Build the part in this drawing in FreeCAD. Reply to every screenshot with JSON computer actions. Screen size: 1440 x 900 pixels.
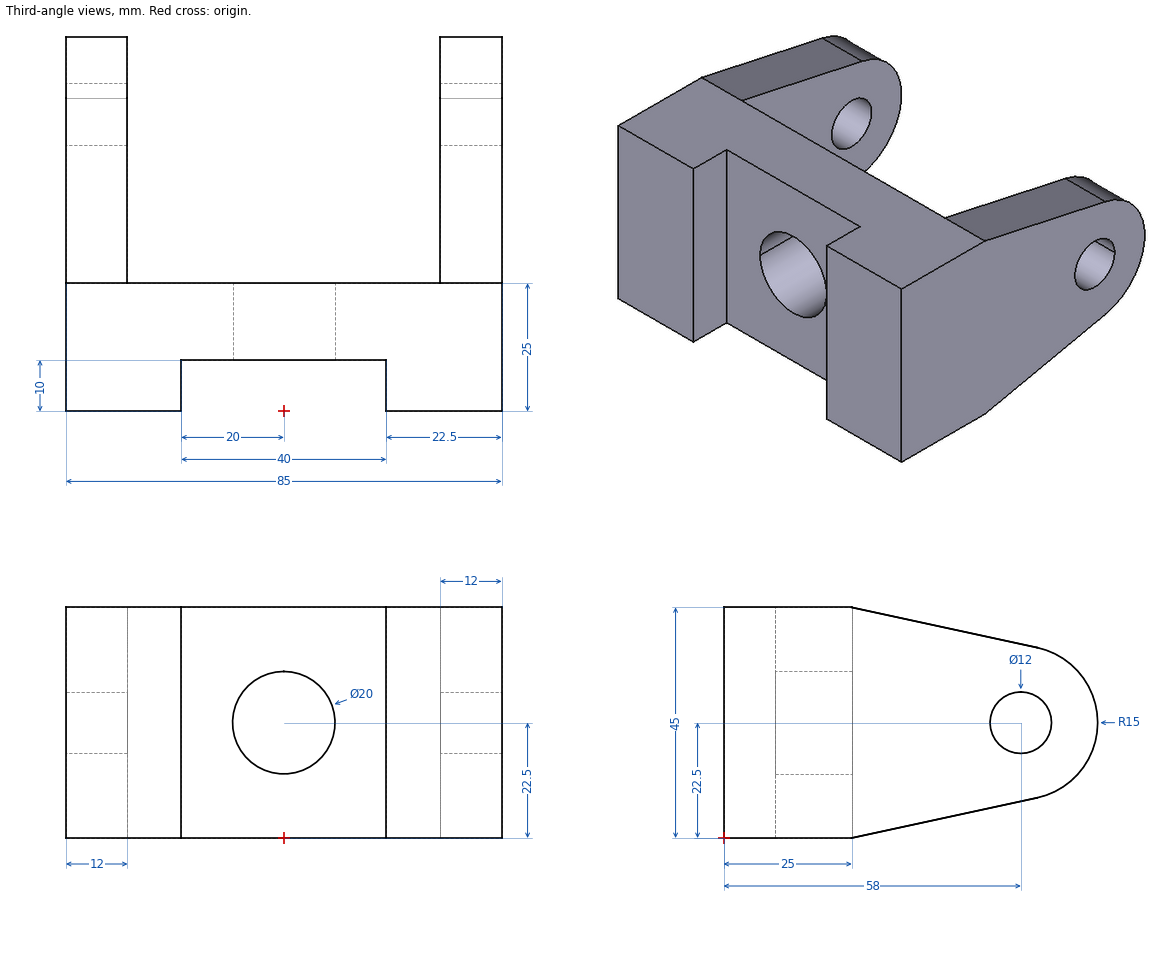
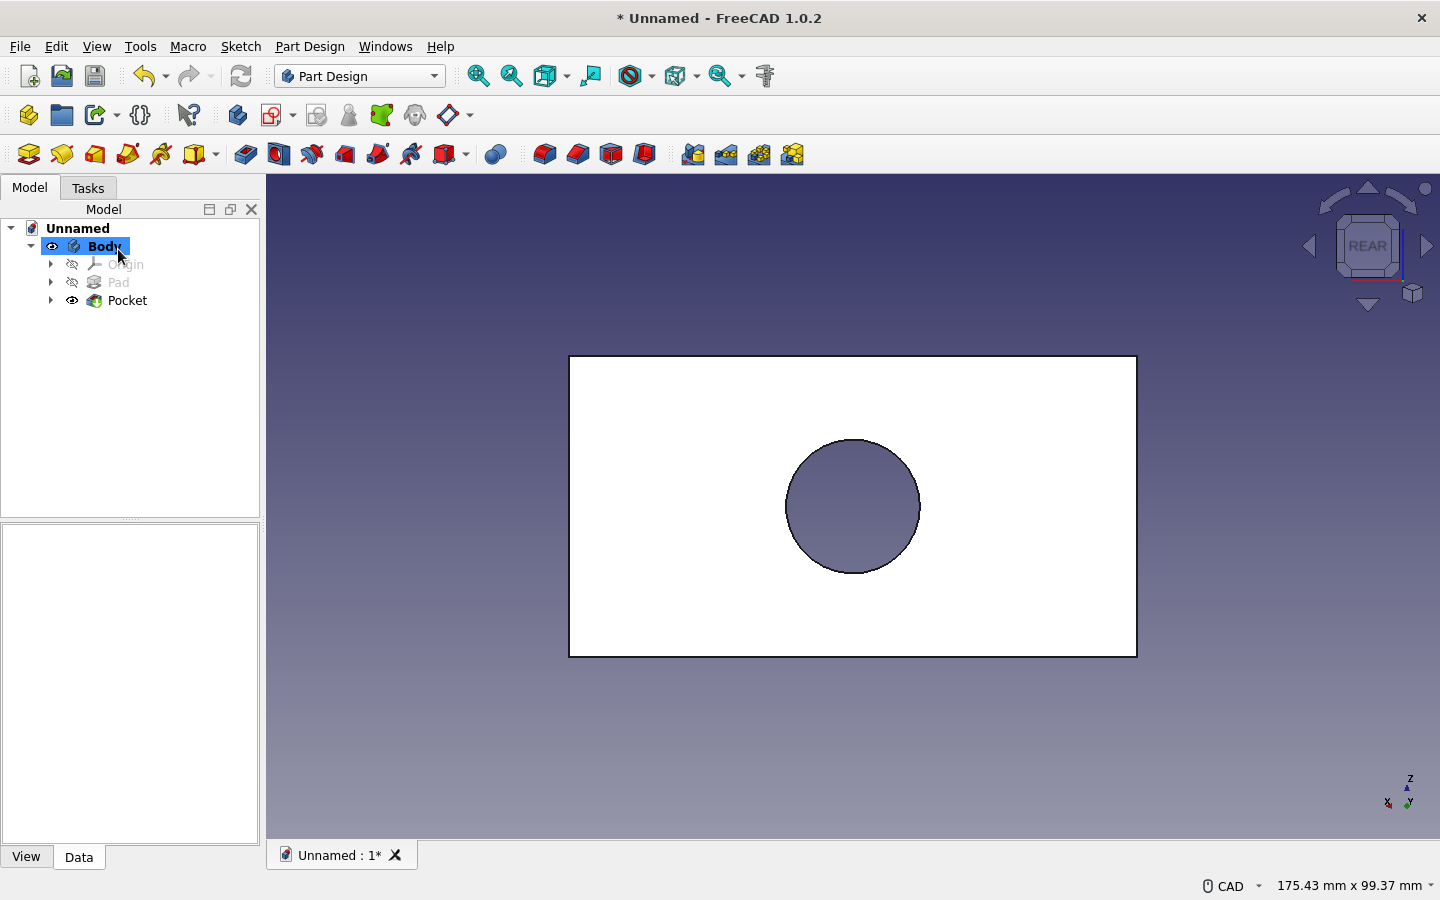
{"action": "key", "text": "6"}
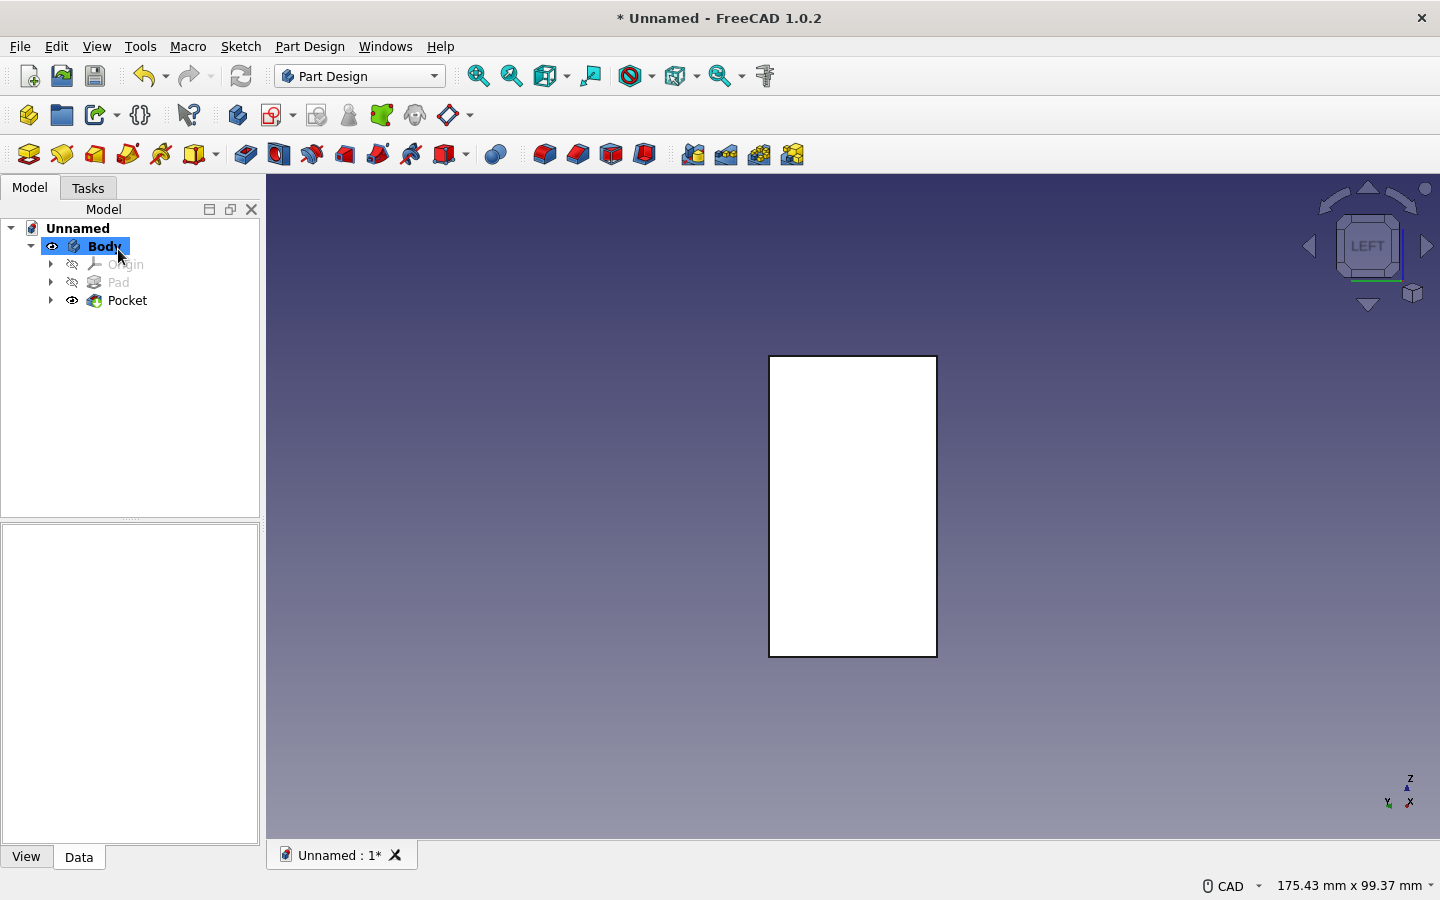
{"action": "left_click", "coordinate": [853, 462]}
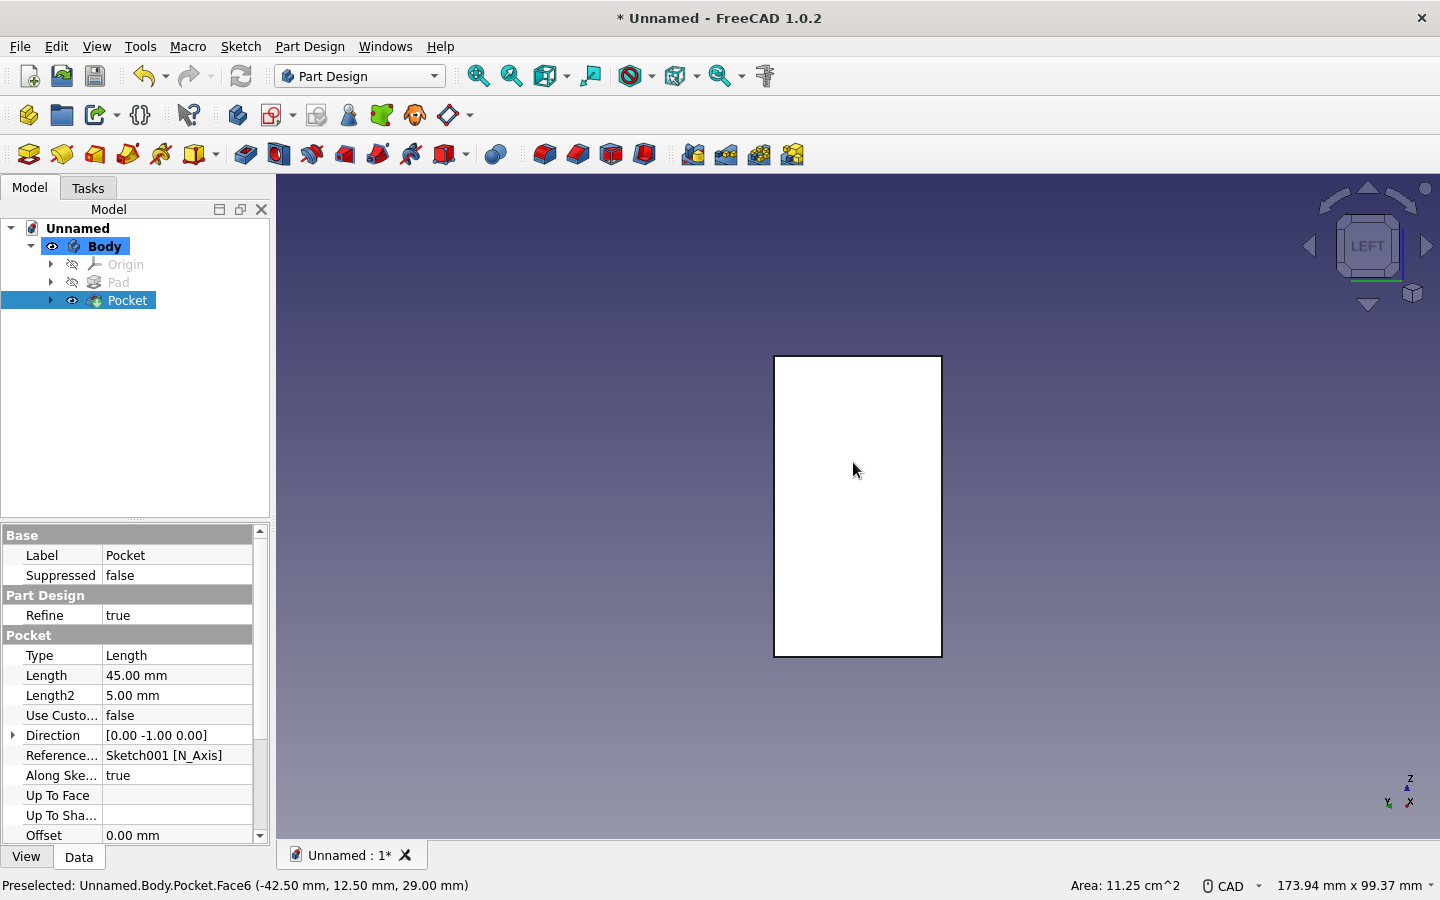
{"action": "left_click", "coordinate": [270, 116]}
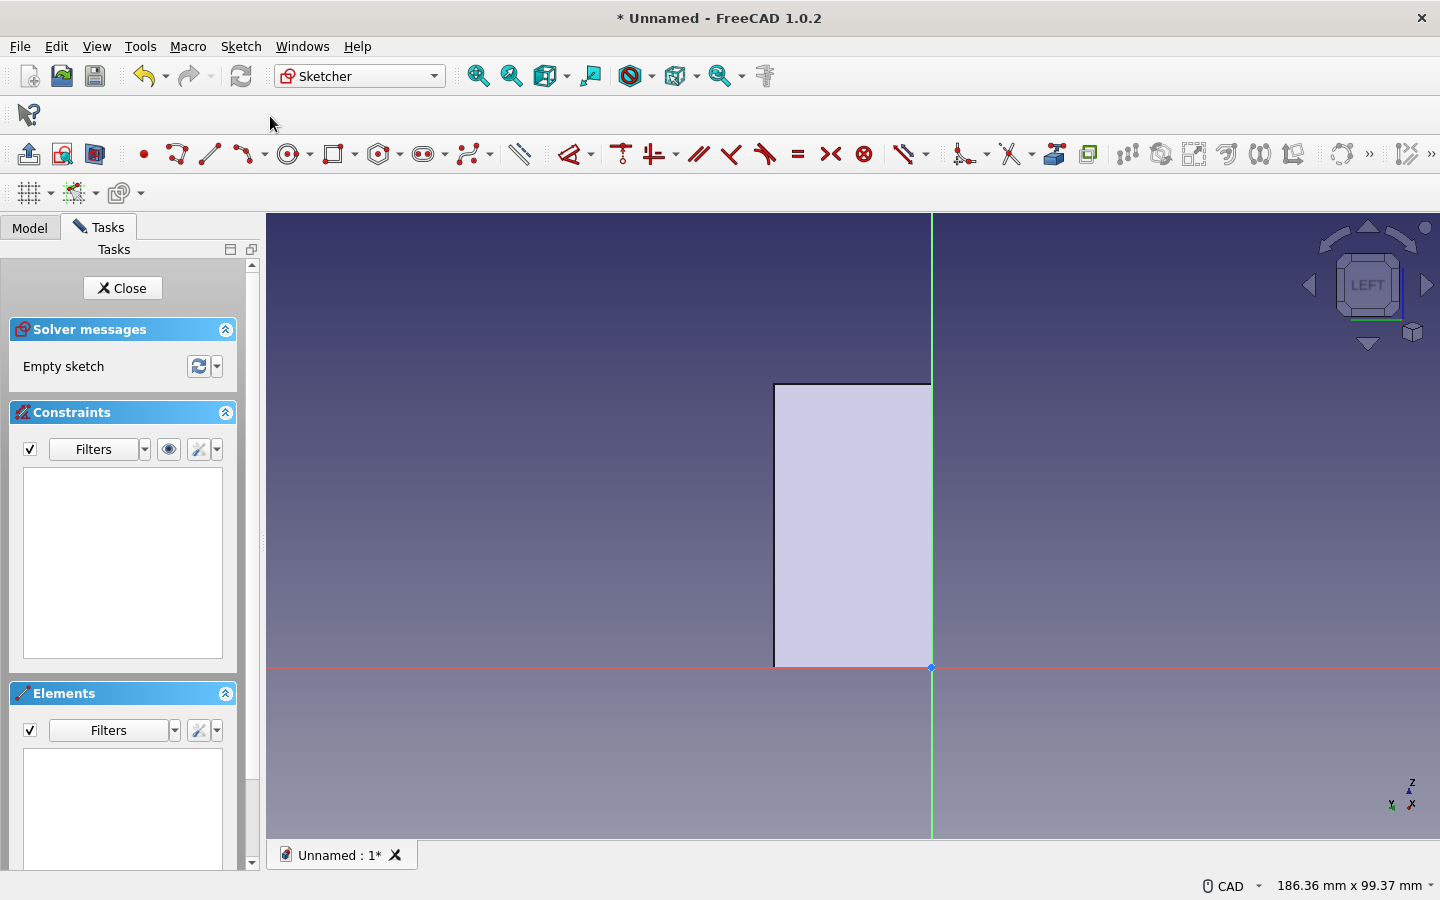
{"action": "scroll", "coordinate": [534, 526], "scroll_direction": "up", "scroll_amount": 2}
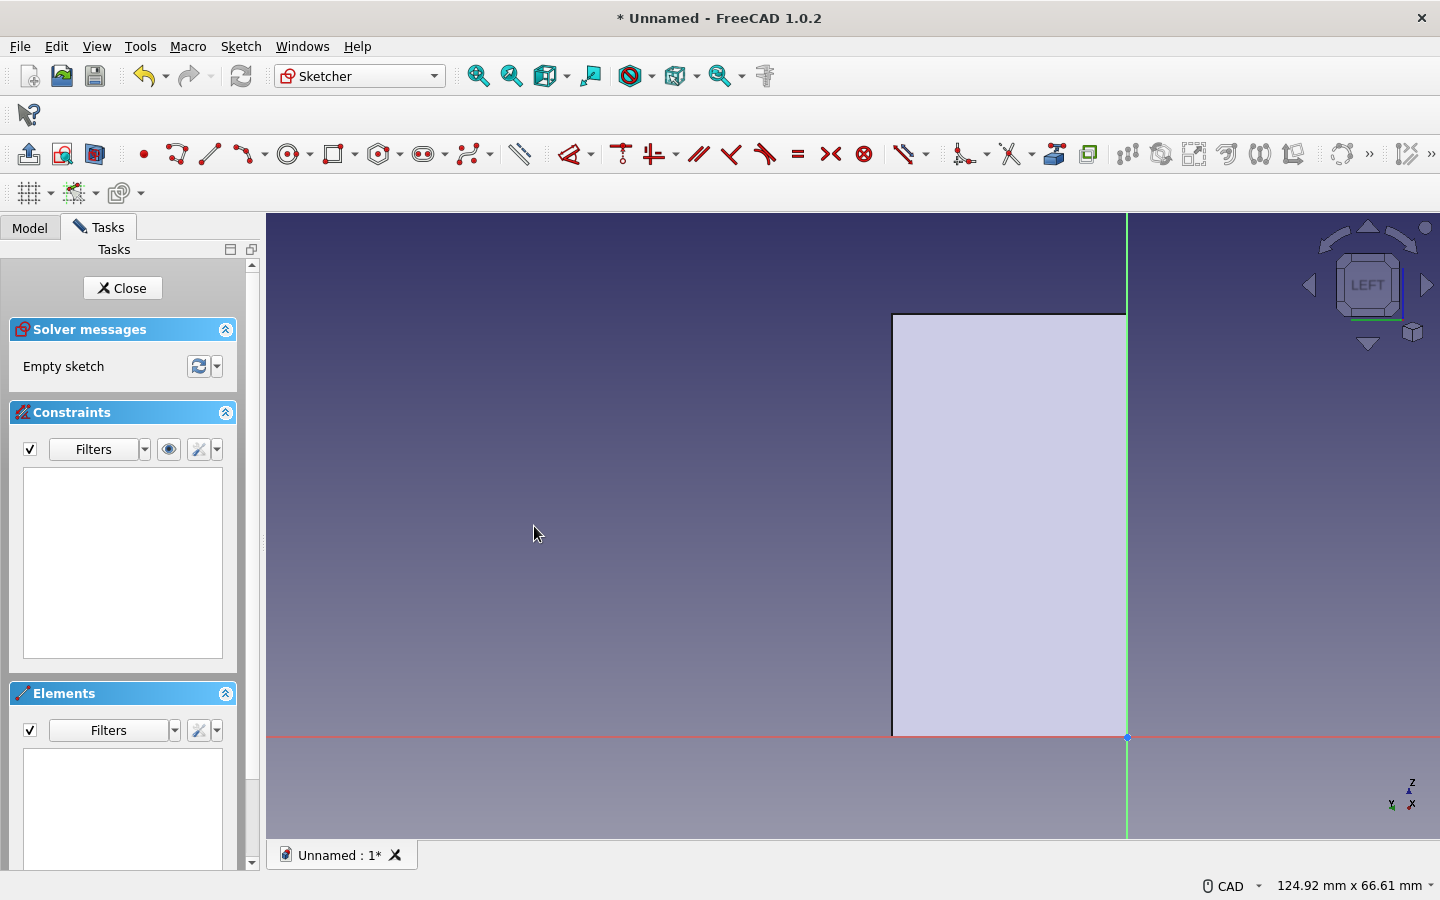
{"action": "left_click", "coordinate": [177, 154]}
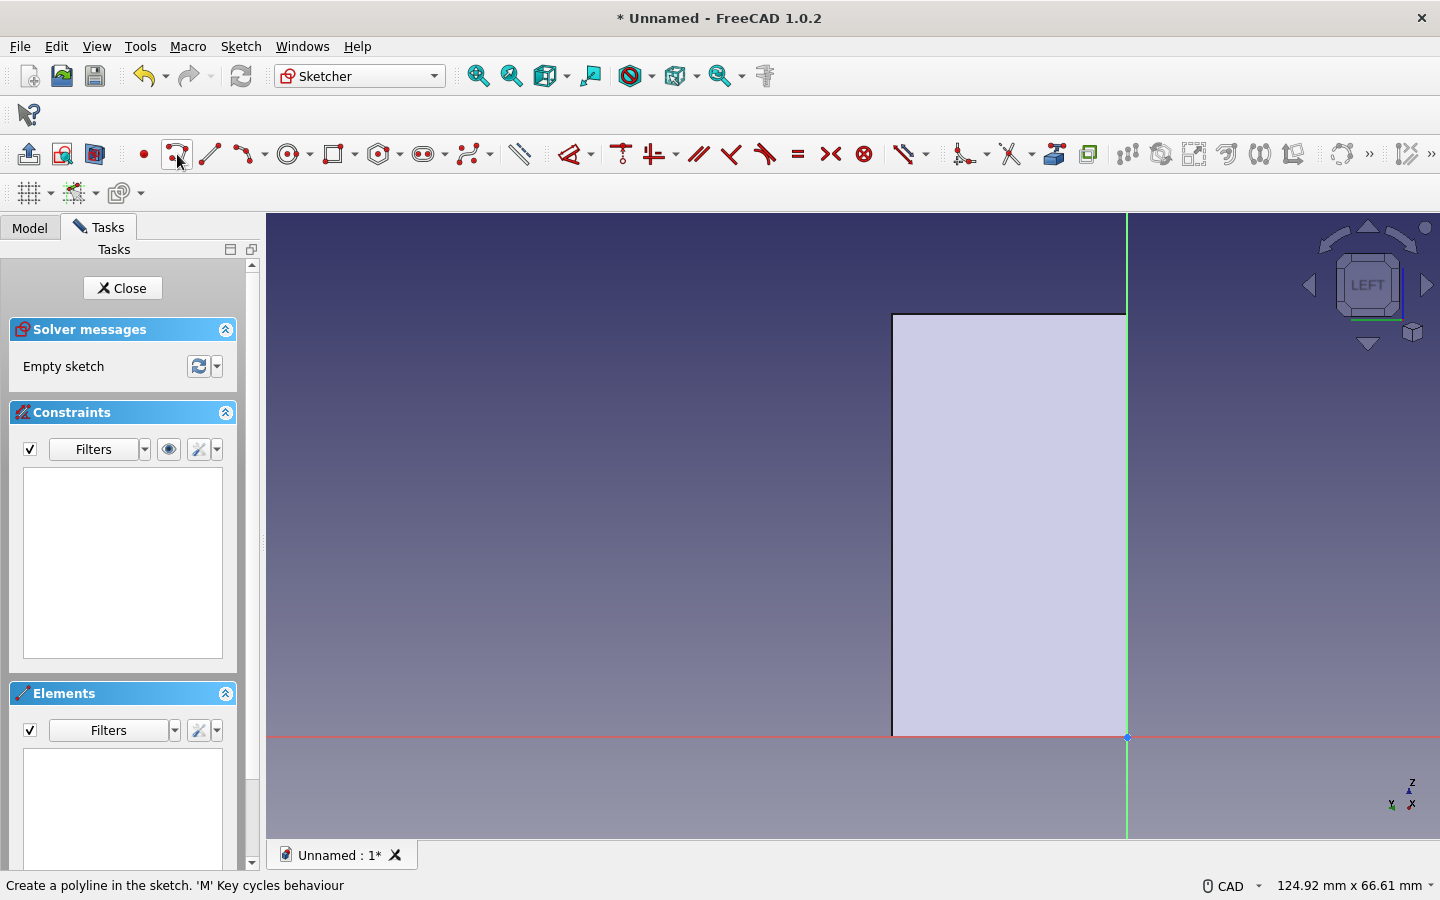
{"action": "left_click", "coordinate": [552, 664]}
{"action": "left_click", "coordinate": [892, 737]}
{"action": "left_click", "coordinate": [892, 314]}
{"action": "left_click", "coordinate": [552, 388]}
{"action": "right_click", "coordinate": [552, 388]}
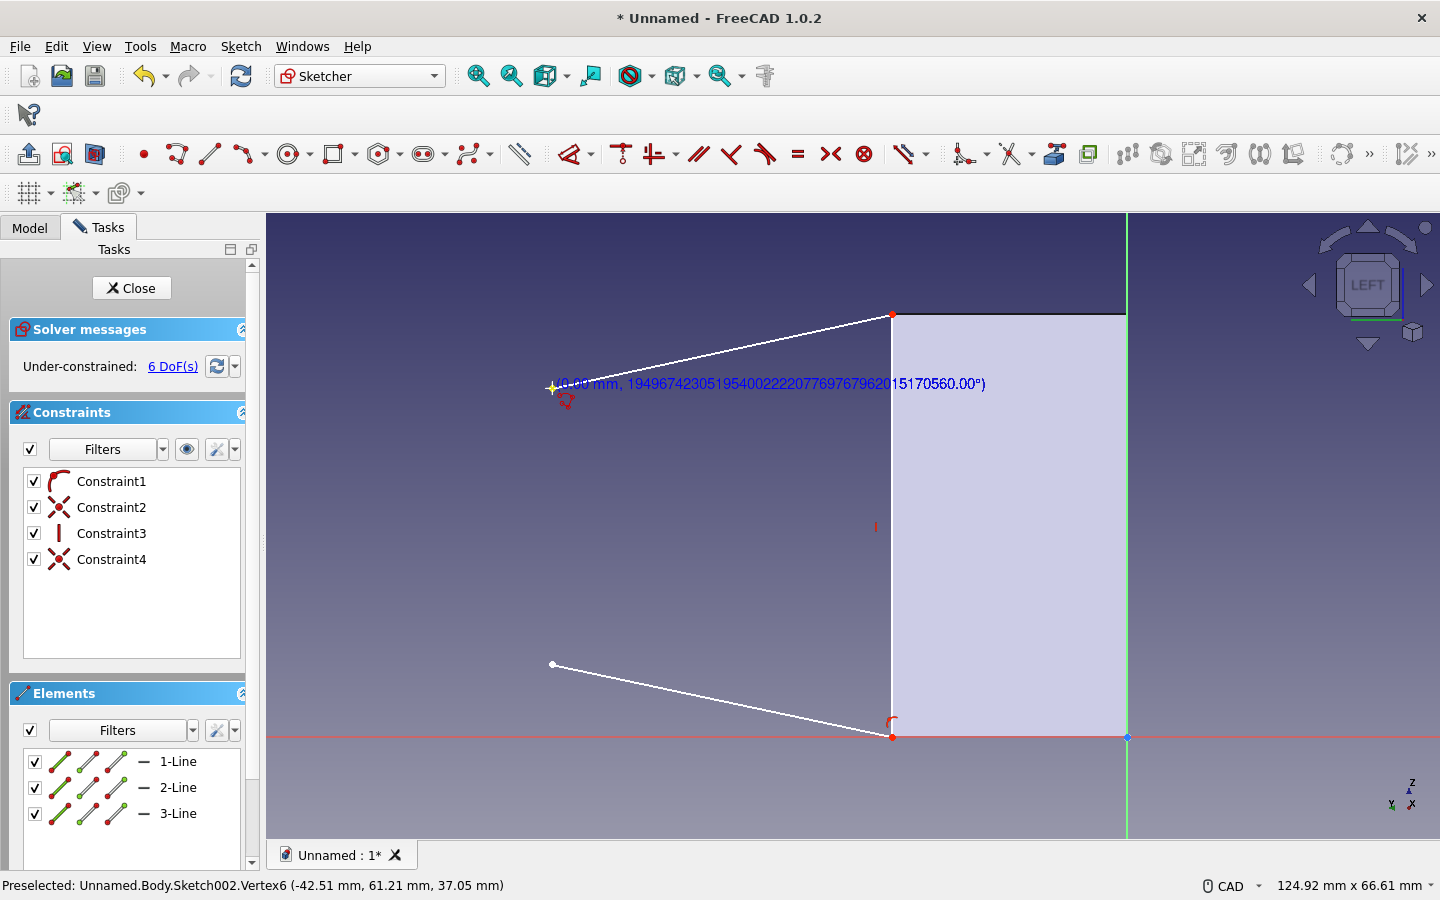
{"action": "left_click", "coordinate": [242, 154]}